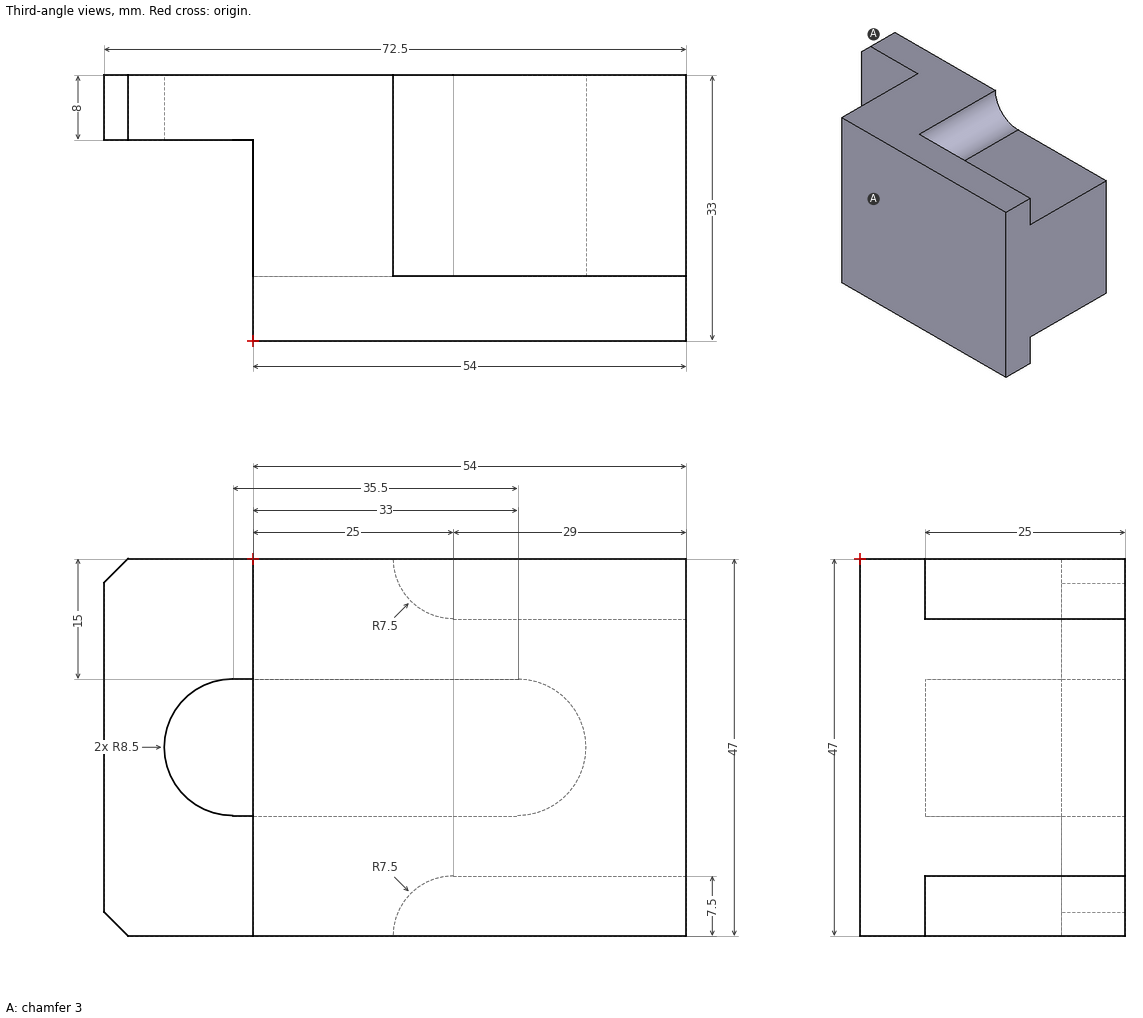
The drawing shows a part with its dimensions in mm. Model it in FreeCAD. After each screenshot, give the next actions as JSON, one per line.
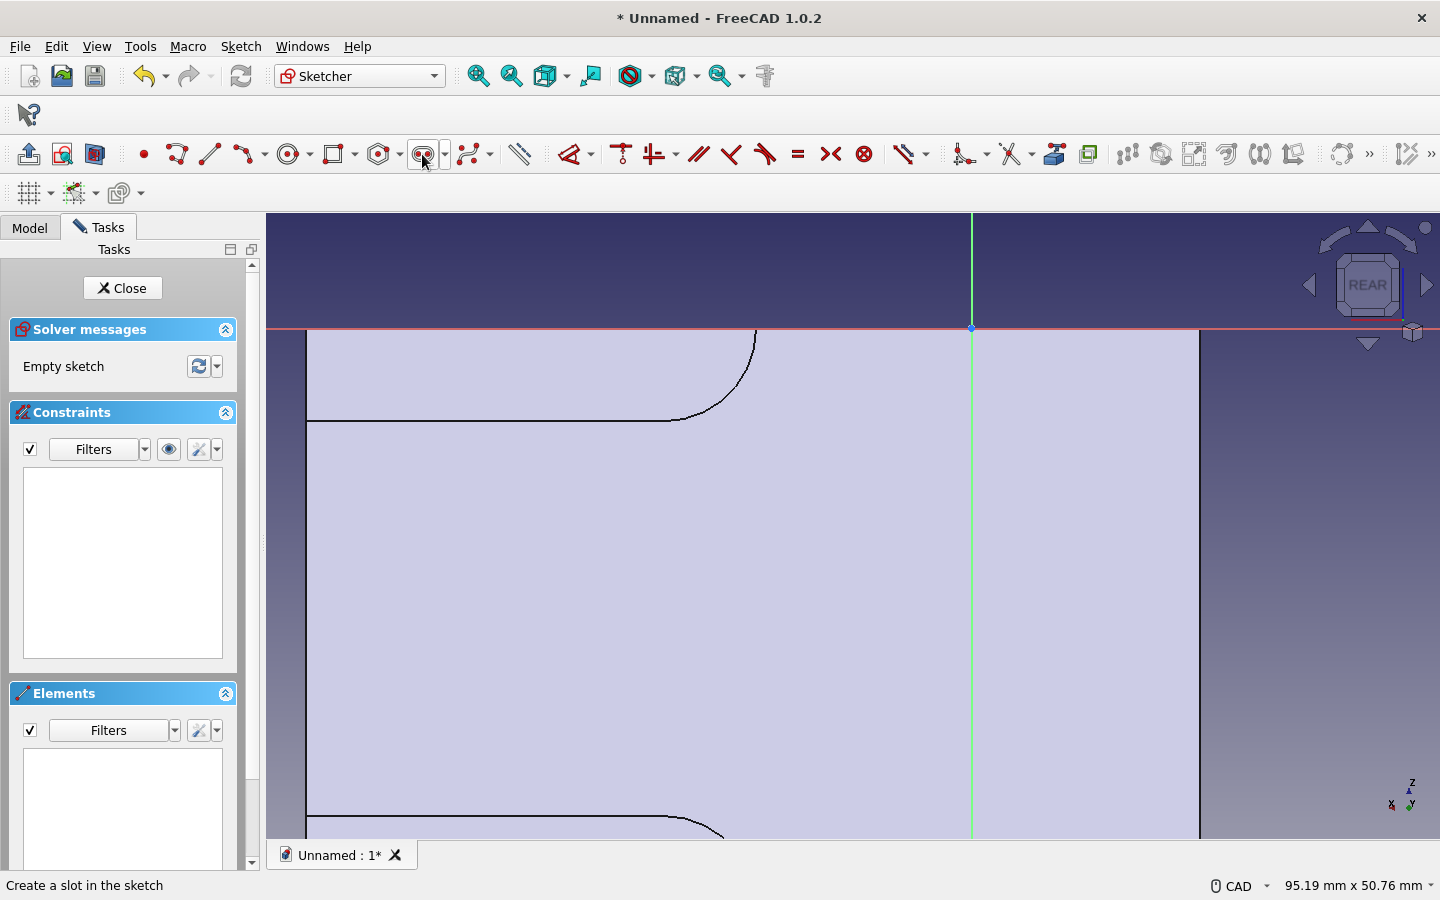
{"action": "left_click", "coordinate": [565, 619]}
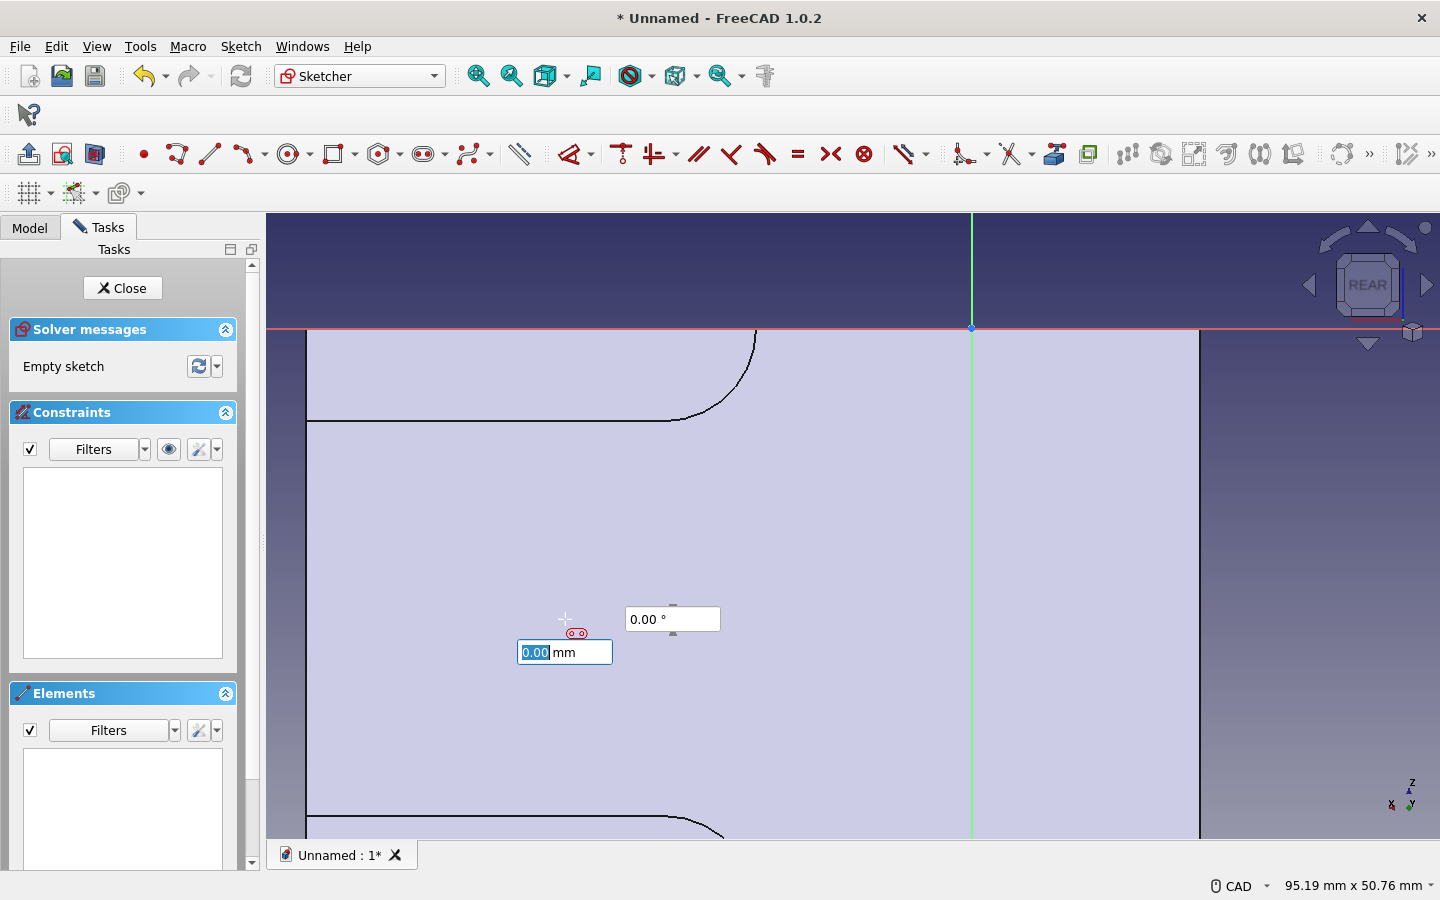
{"action": "left_click", "coordinate": [1003, 619]}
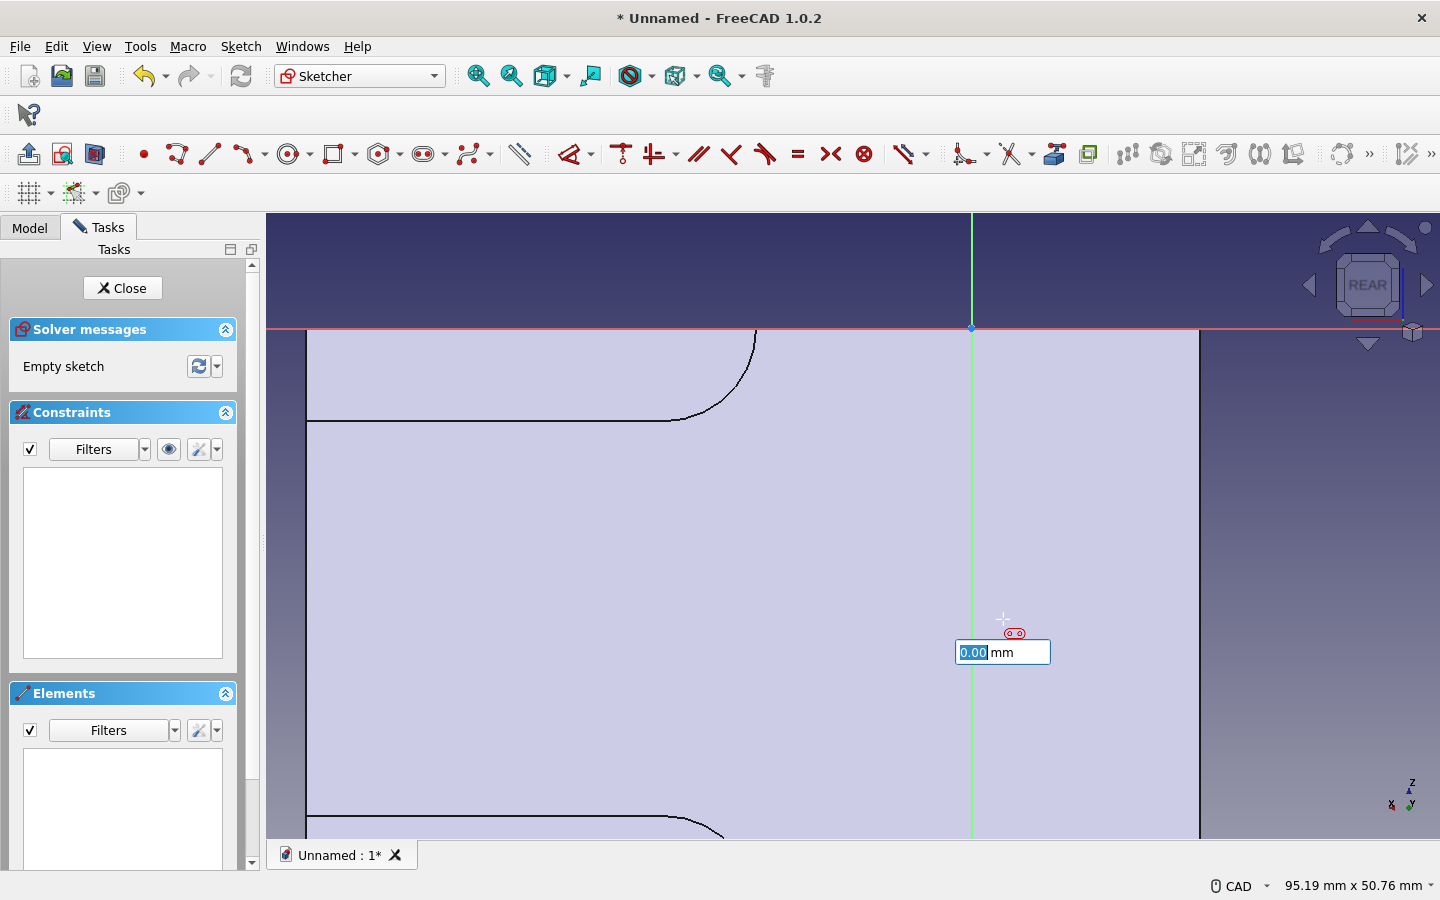
{"action": "left_click", "coordinate": [784, 723]}
{"action": "key", "text": "Escape"}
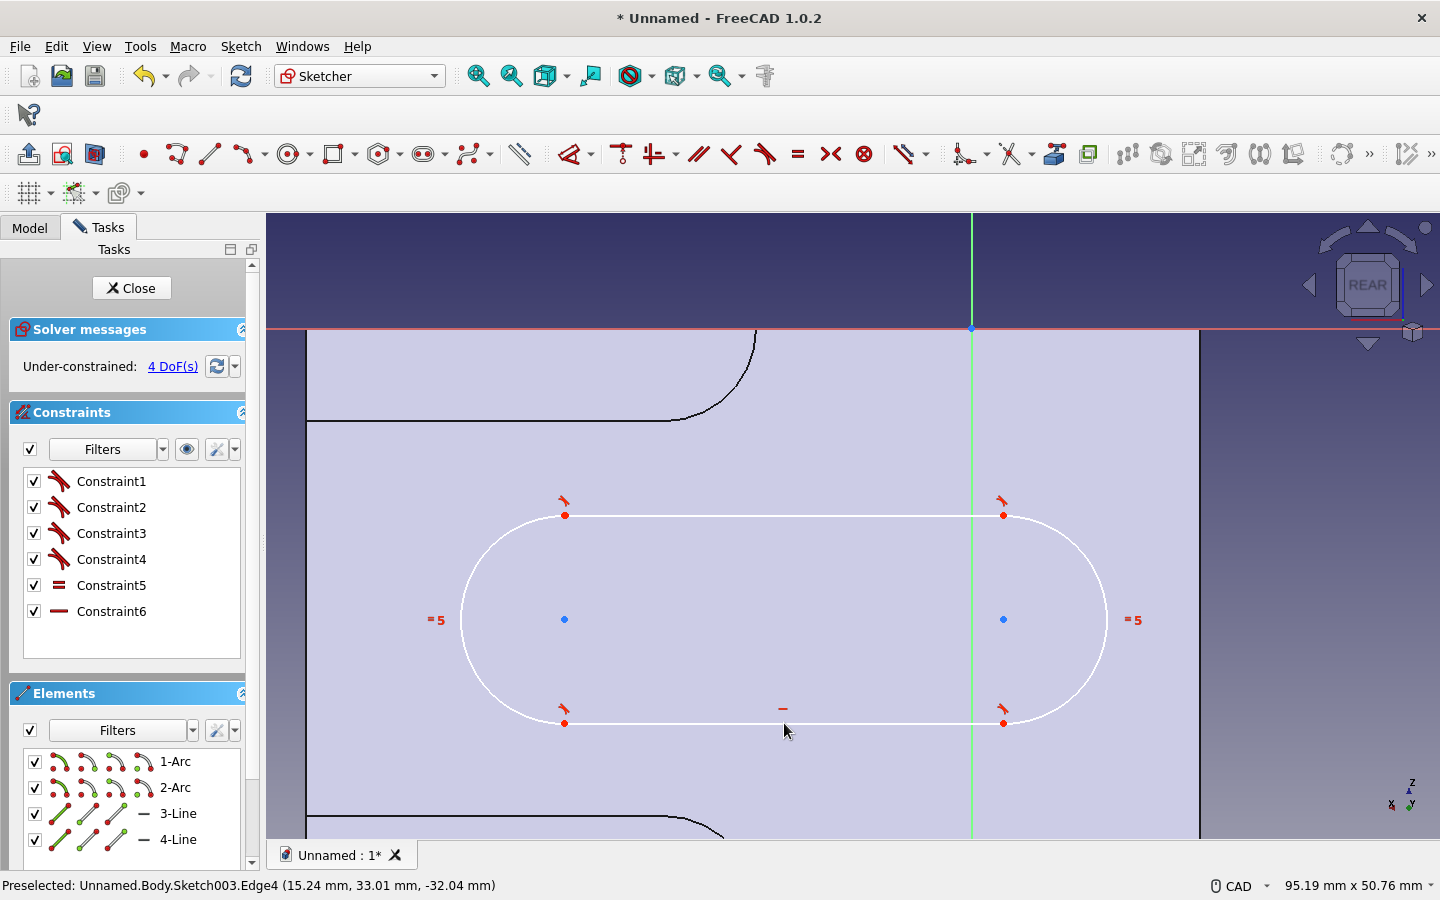
{"action": "key", "text": "d"}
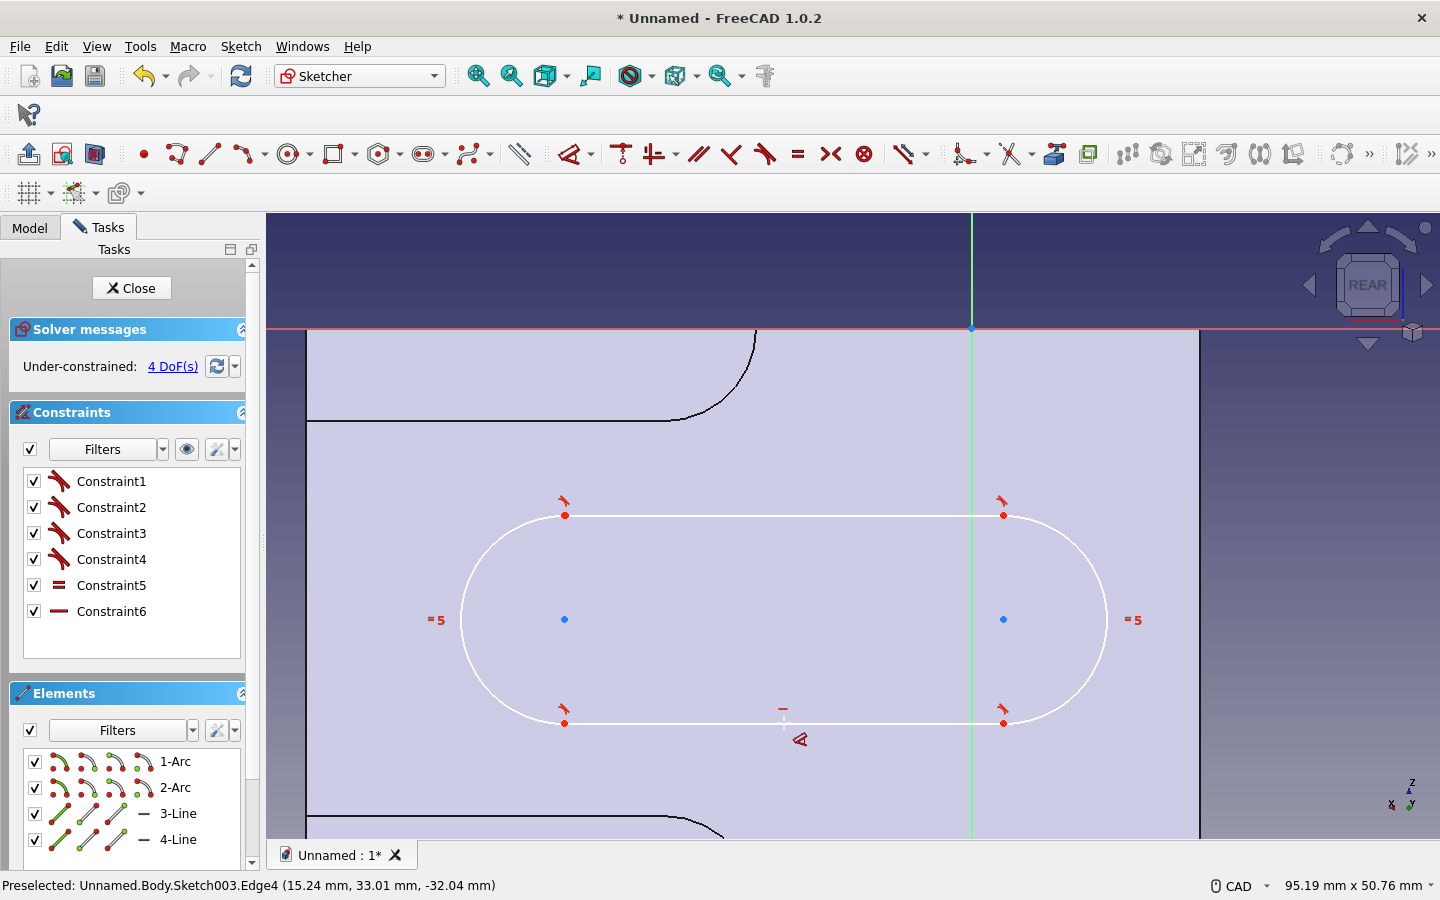
{"action": "left_click", "coordinate": [481, 559]}
{"action": "left_click", "coordinate": [455, 540]}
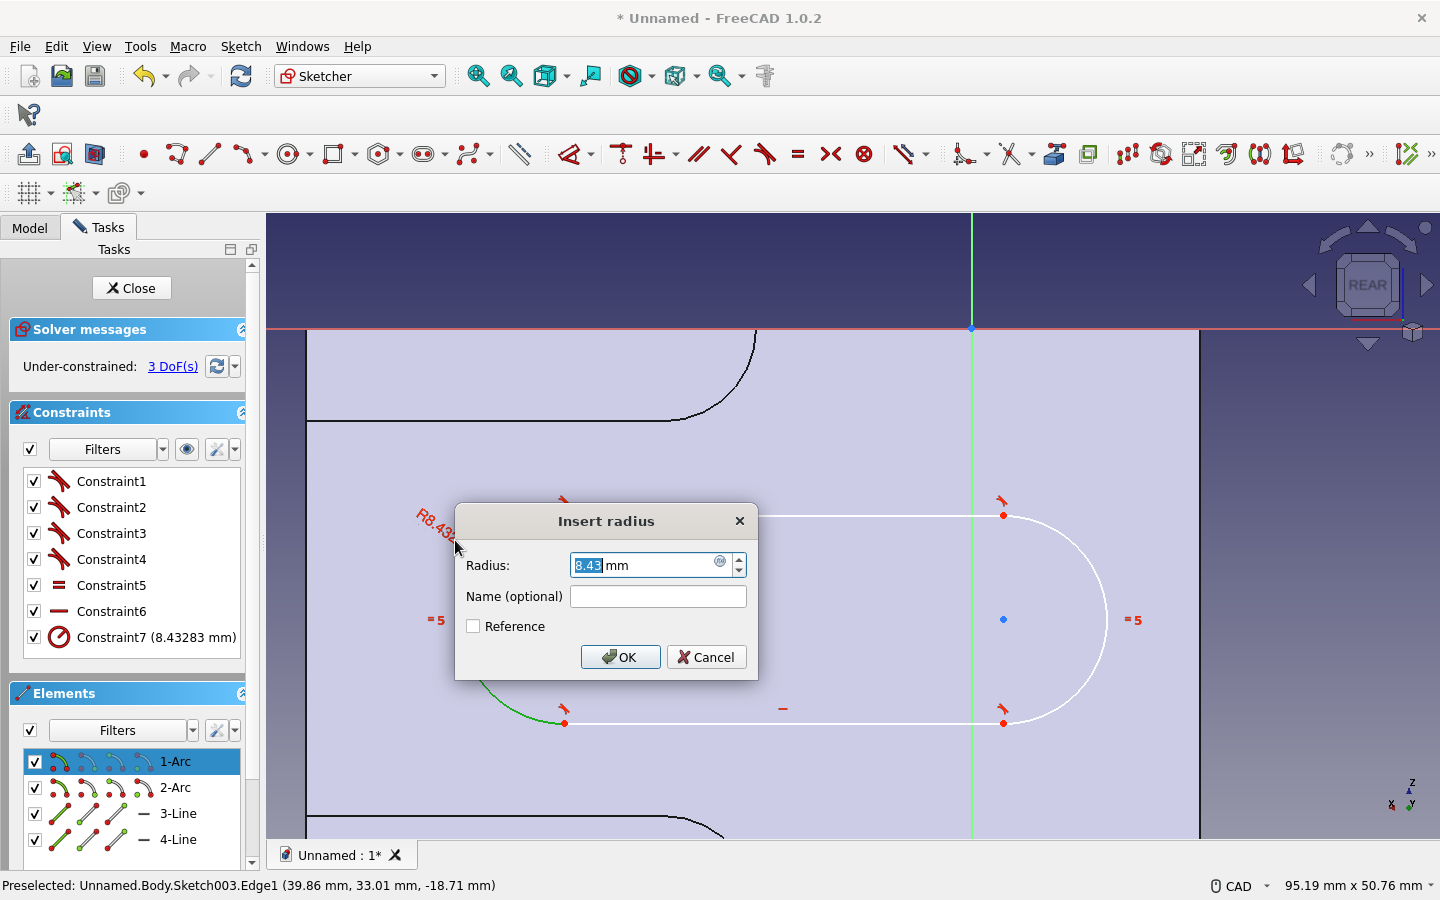
{"action": "type", "text": "8.5"}
{"action": "key", "text": "Return"}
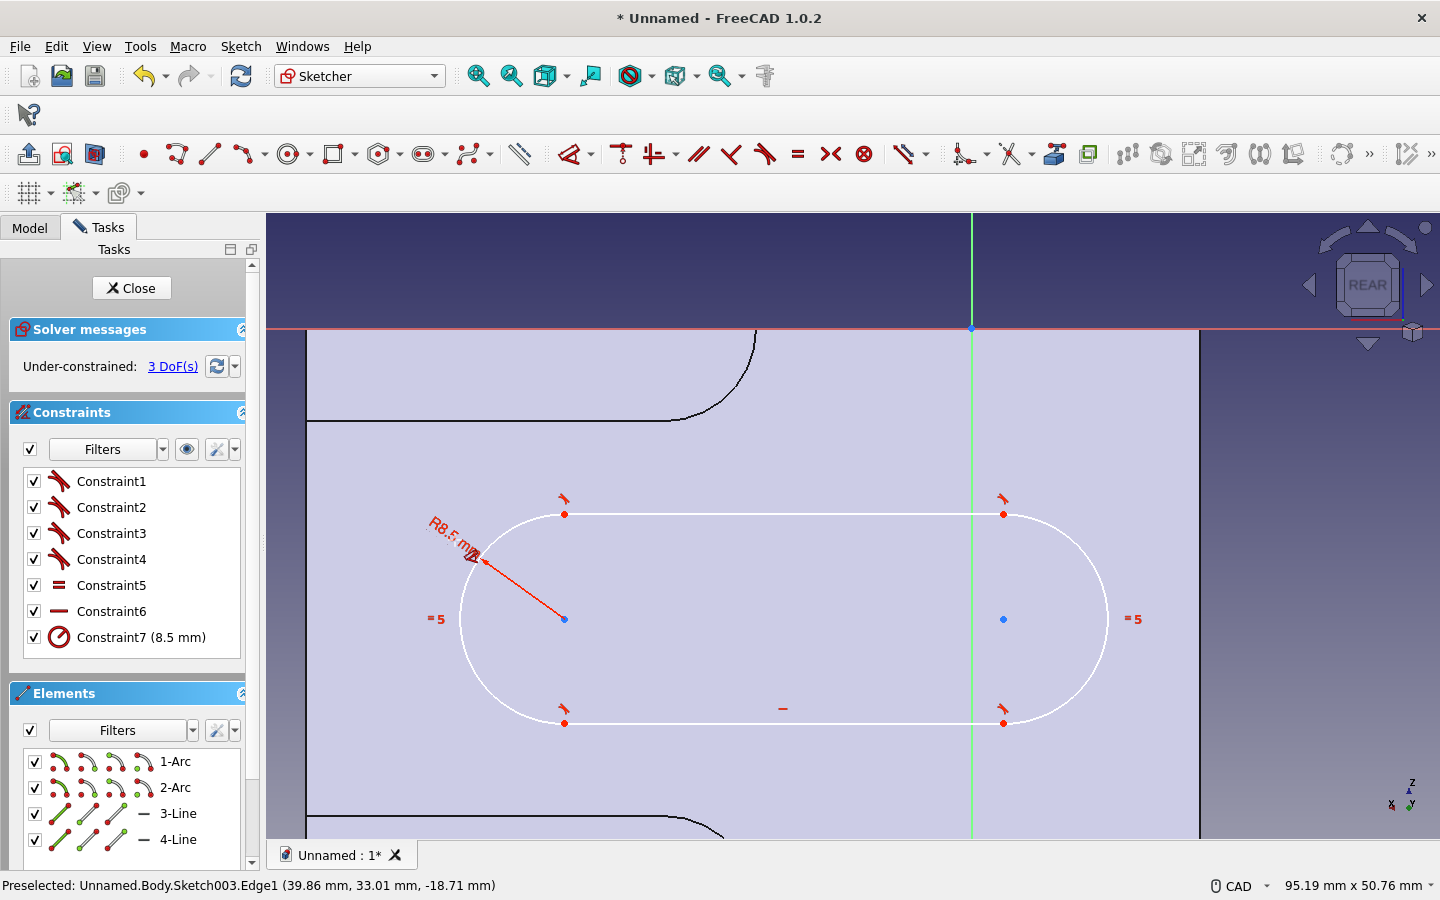
{"action": "left_click", "coordinate": [565, 514]}
{"action": "left_click", "coordinate": [768, 295]}